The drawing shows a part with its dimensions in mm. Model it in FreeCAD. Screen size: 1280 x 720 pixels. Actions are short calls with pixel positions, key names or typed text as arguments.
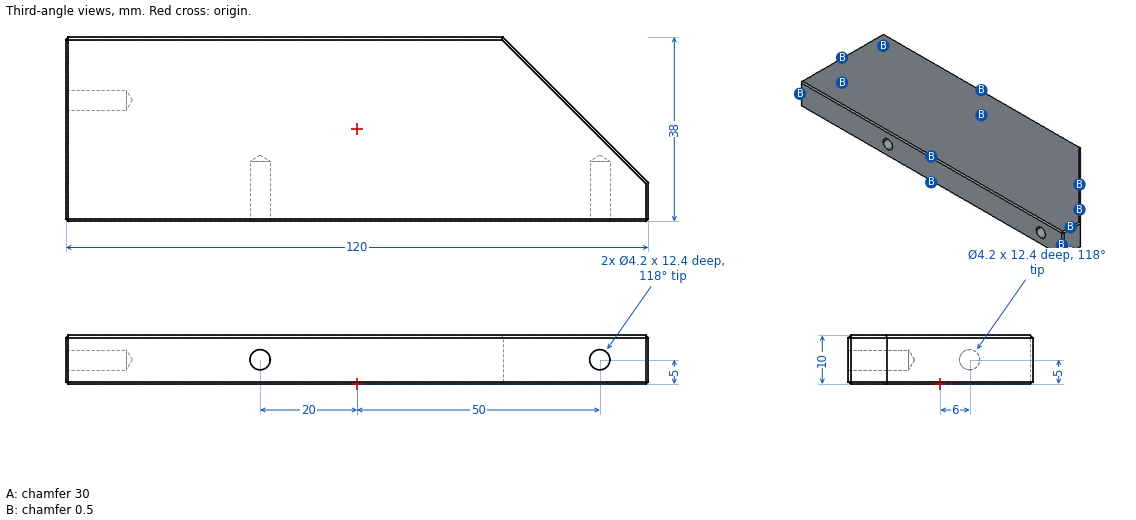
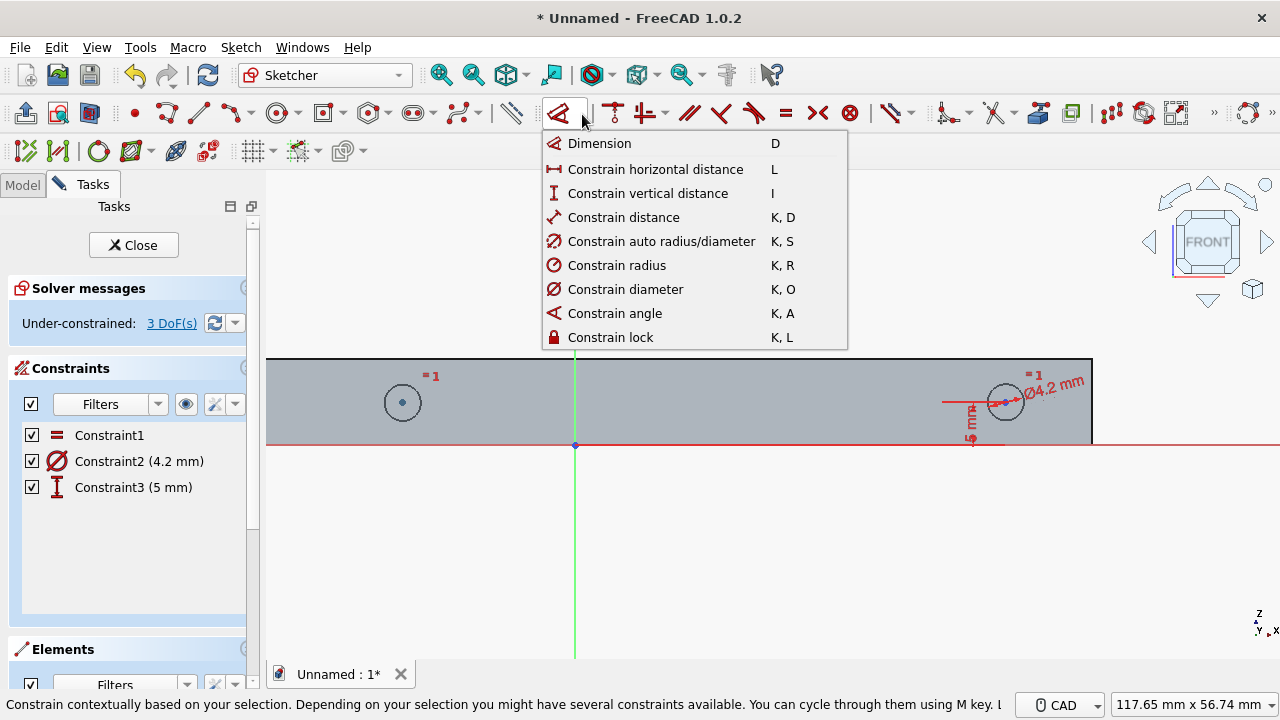
click(695, 193)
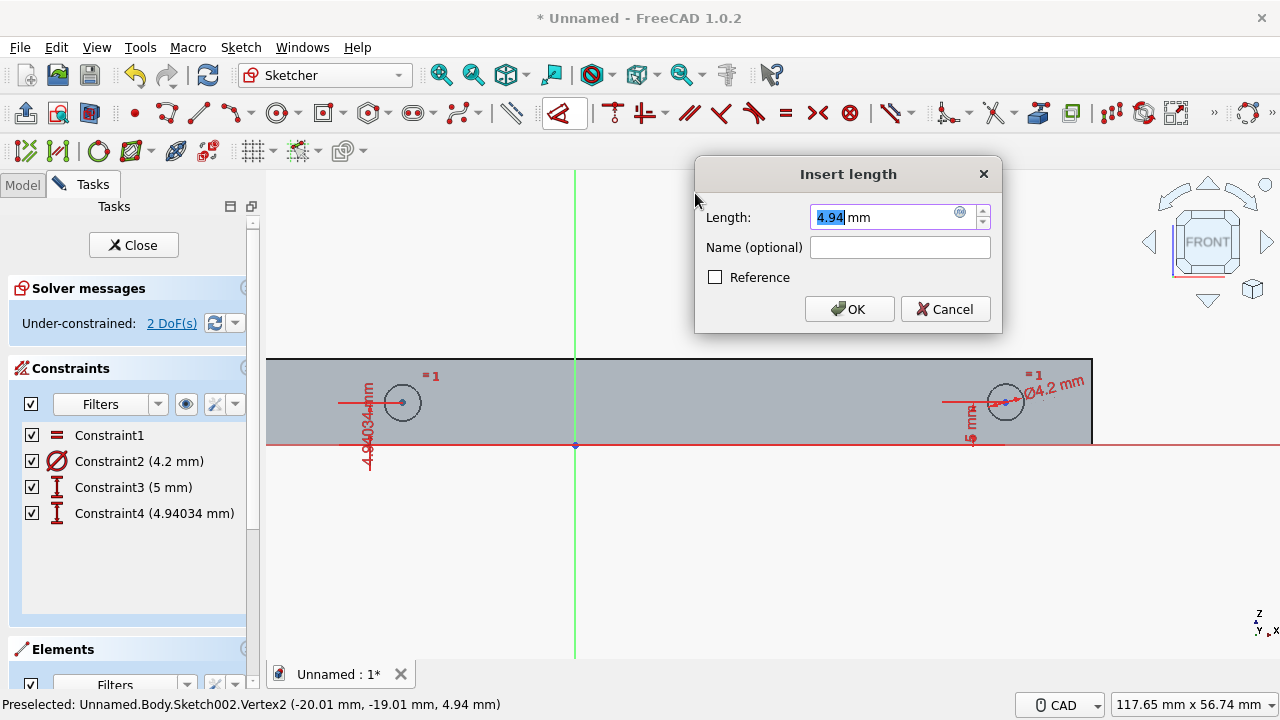
text(5)
key(Return)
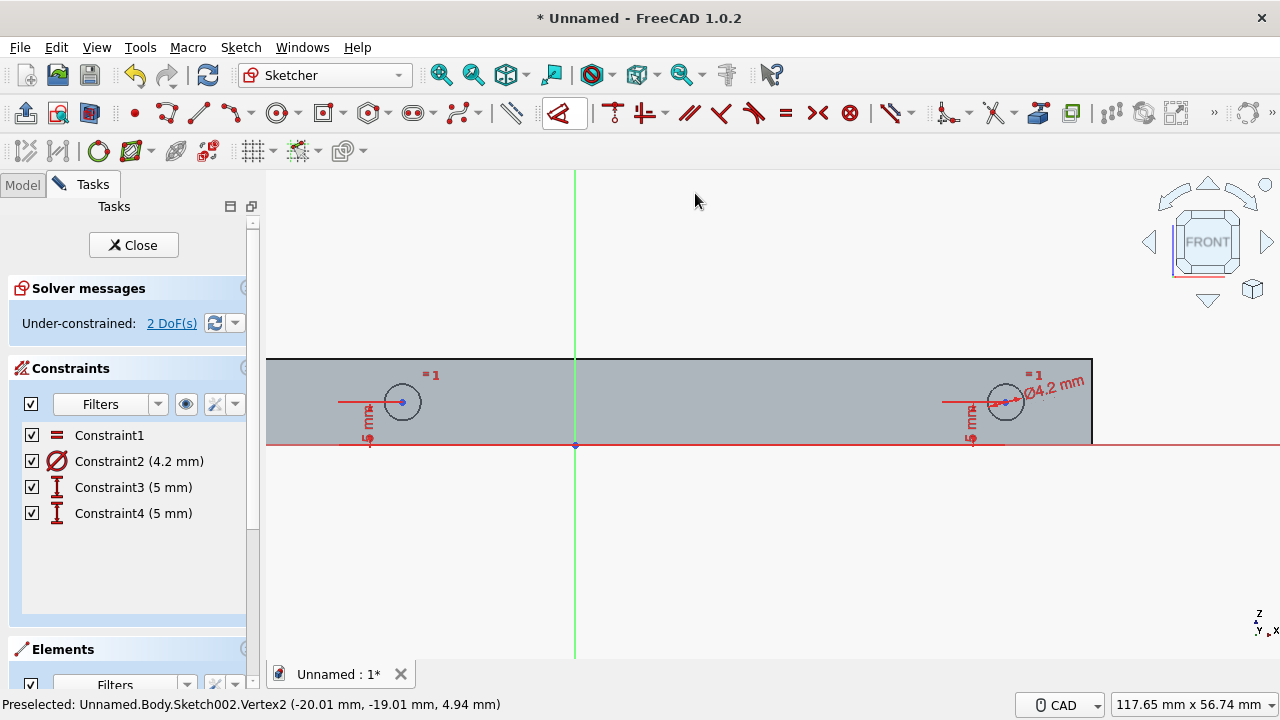
click(1006, 402)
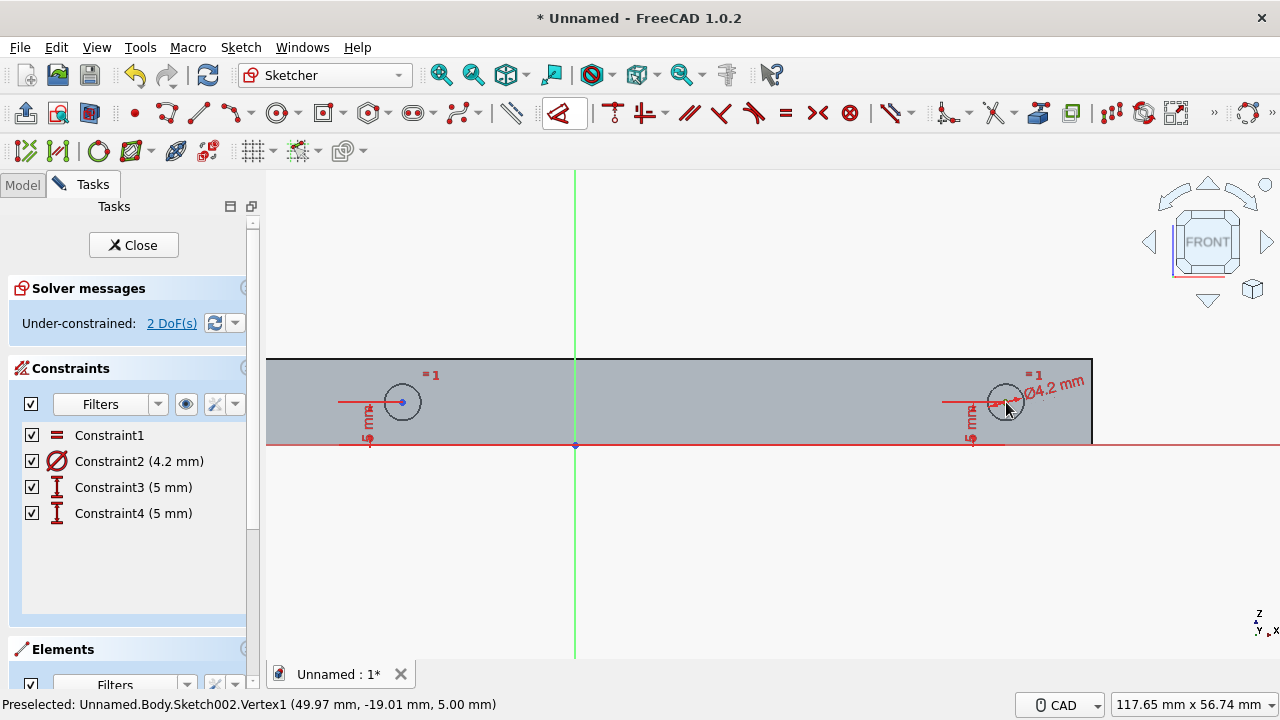
key(l)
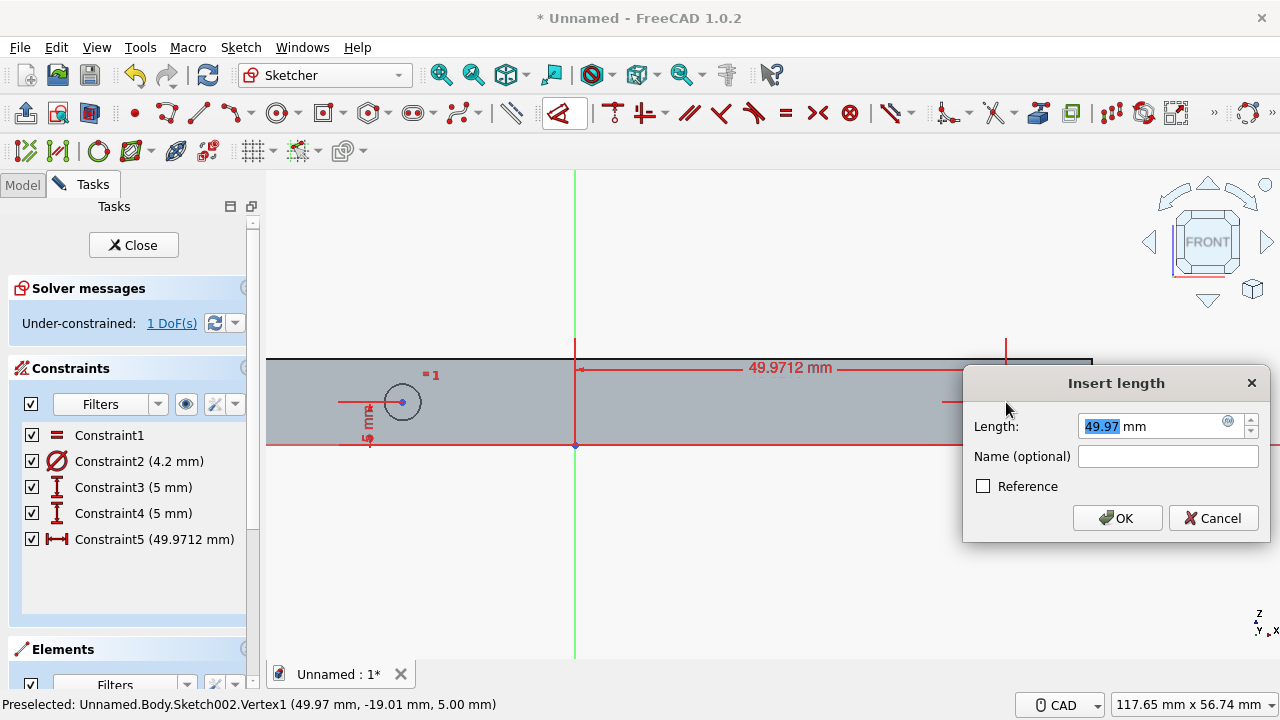
text(50)
key(Return)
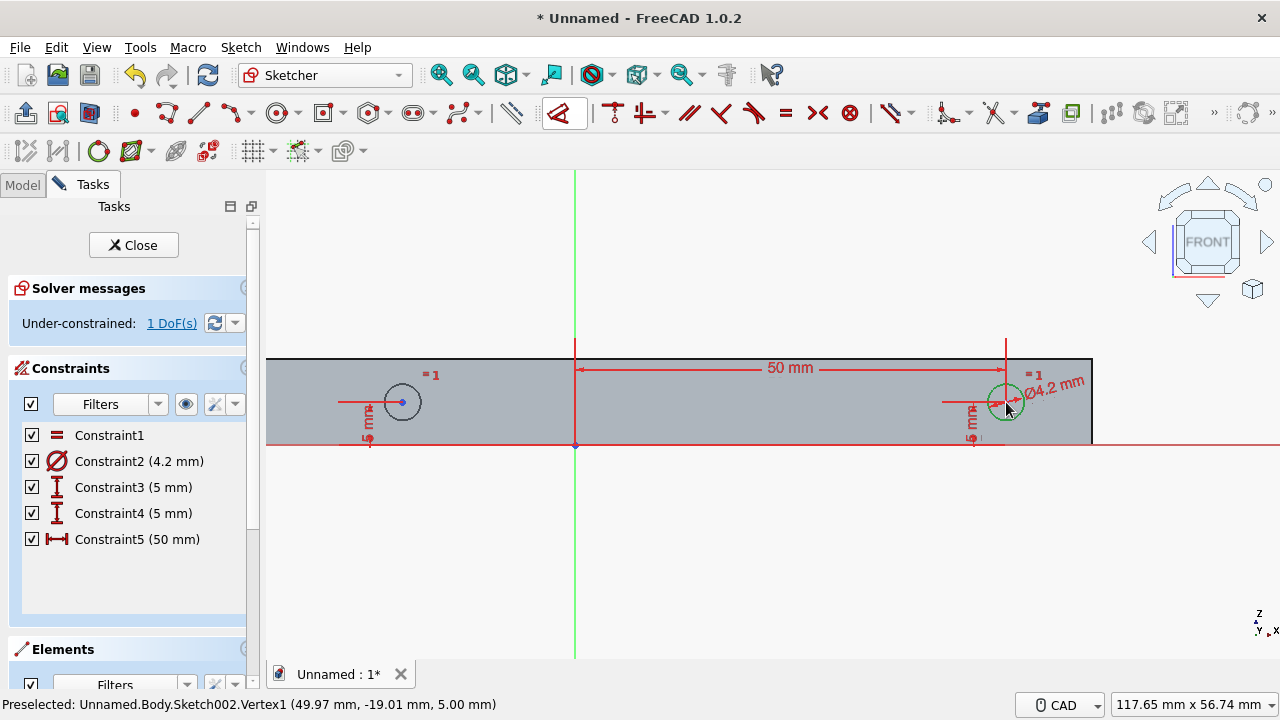
click(403, 402)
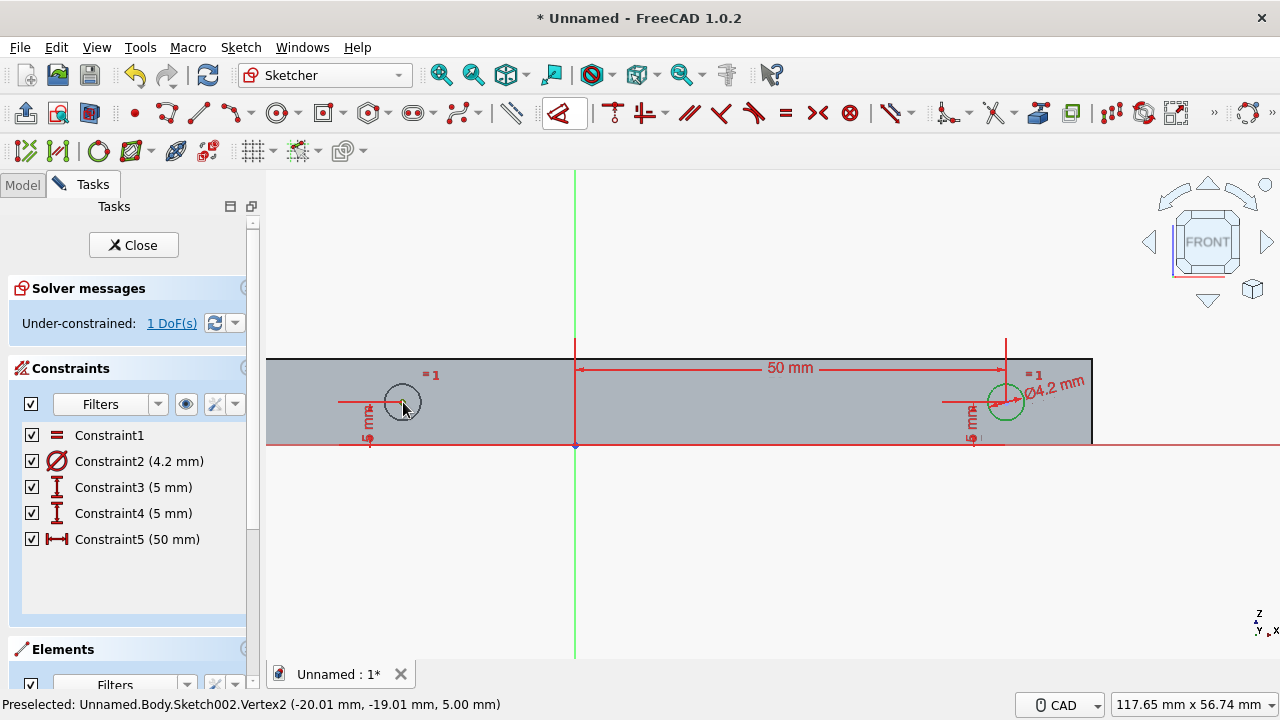
click(582, 114)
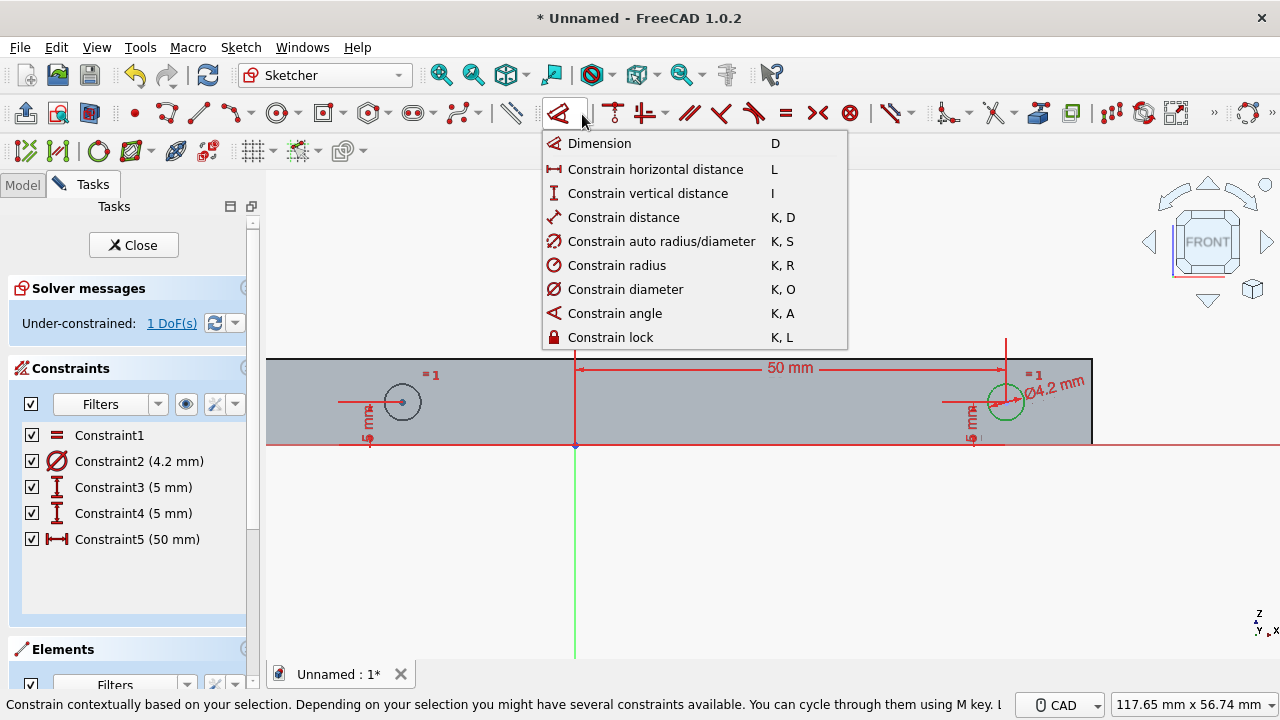
click(695, 169)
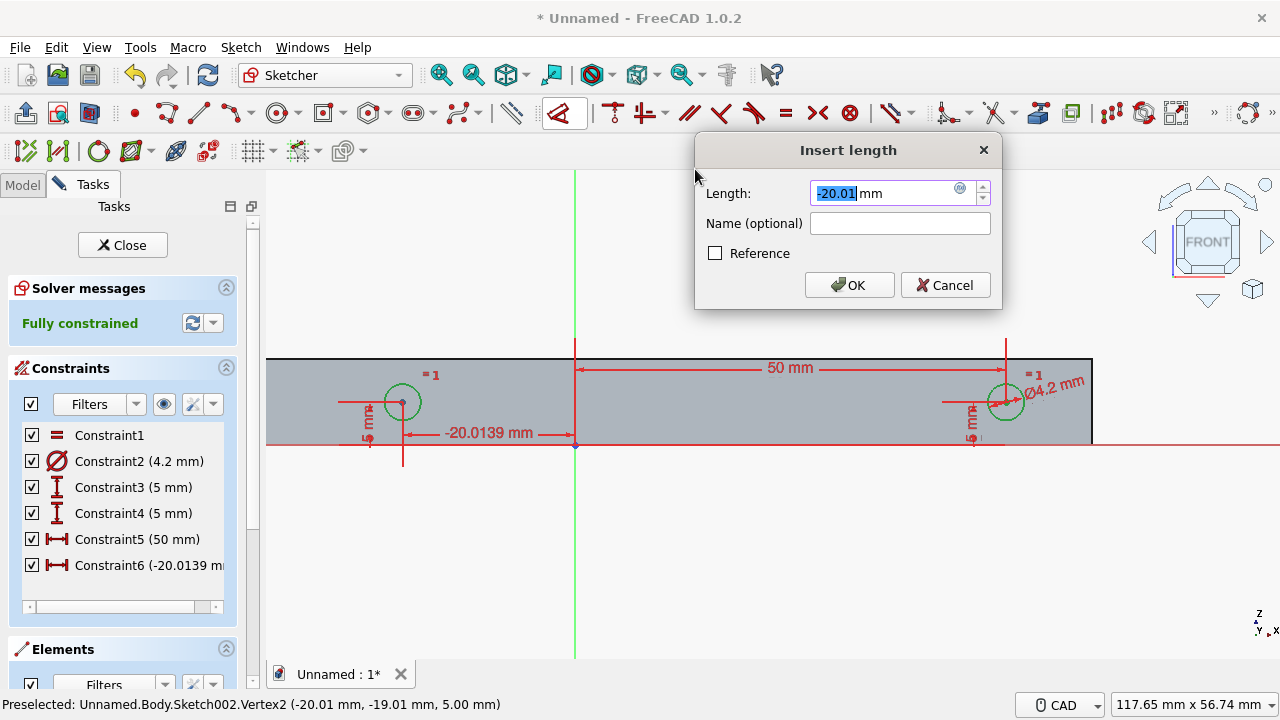
text(-20)
key(Return)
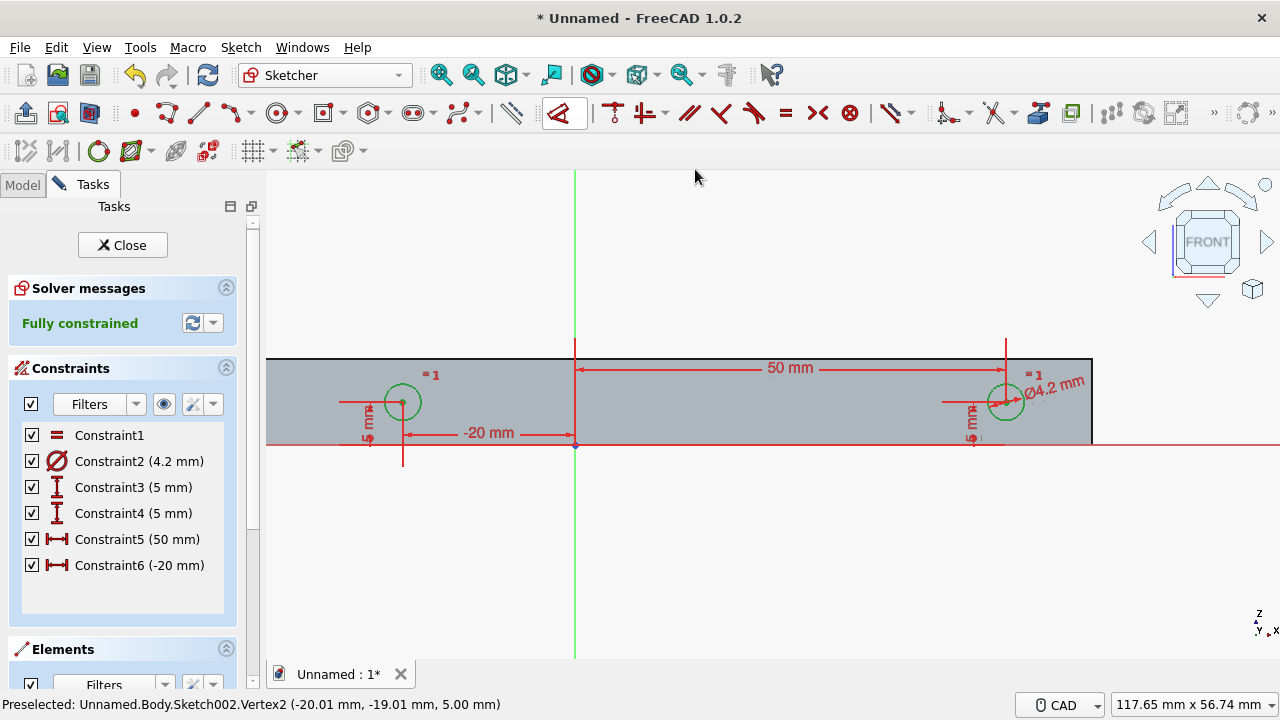
click(123, 245)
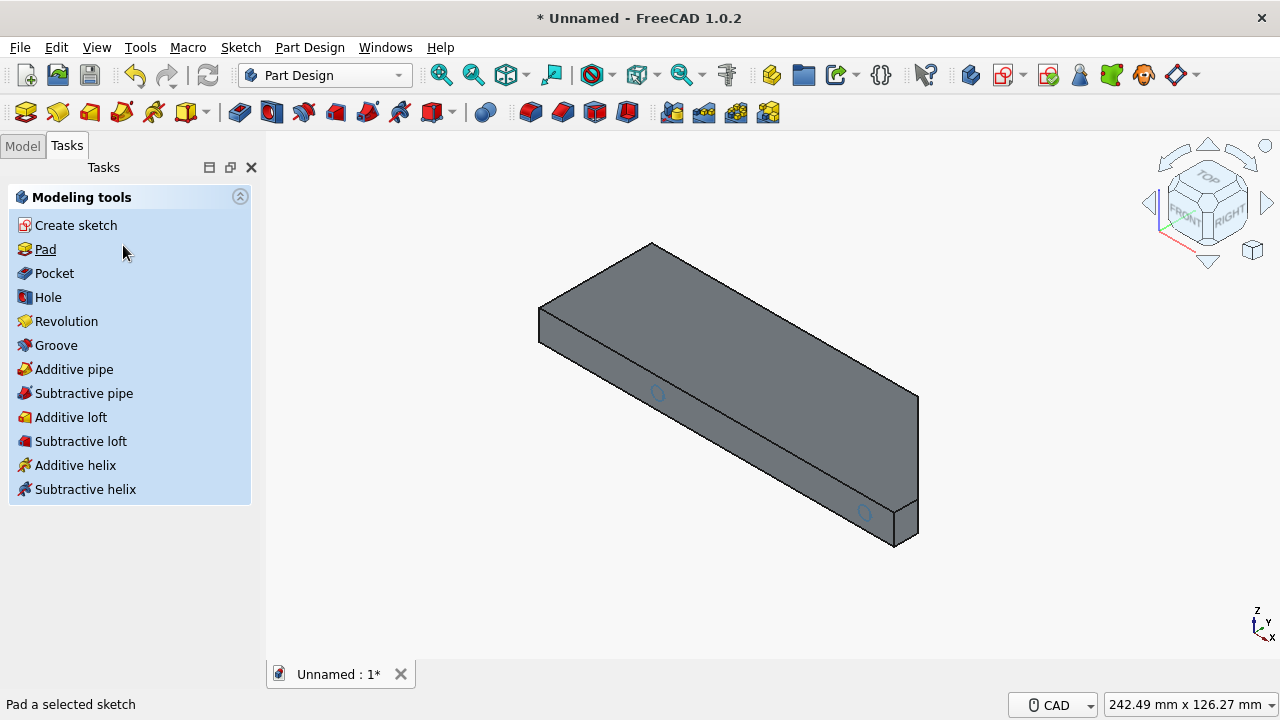
click(272, 112)